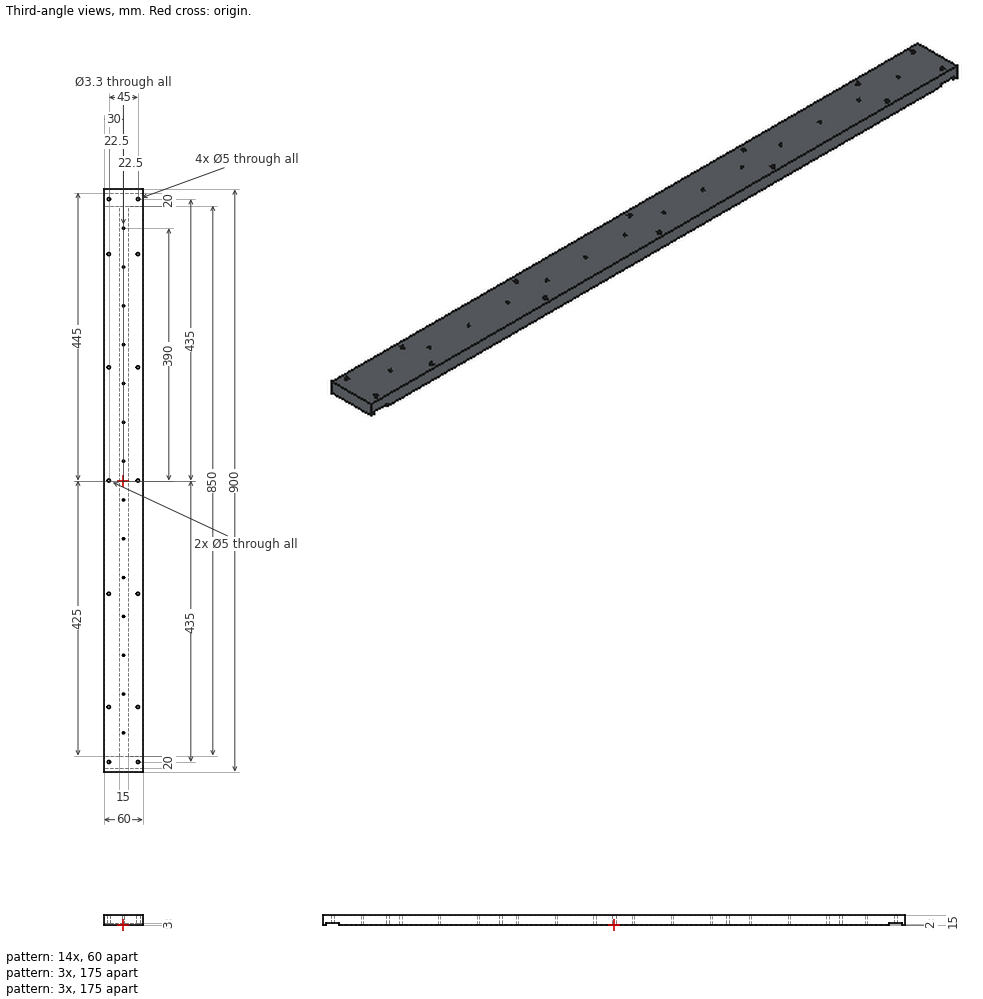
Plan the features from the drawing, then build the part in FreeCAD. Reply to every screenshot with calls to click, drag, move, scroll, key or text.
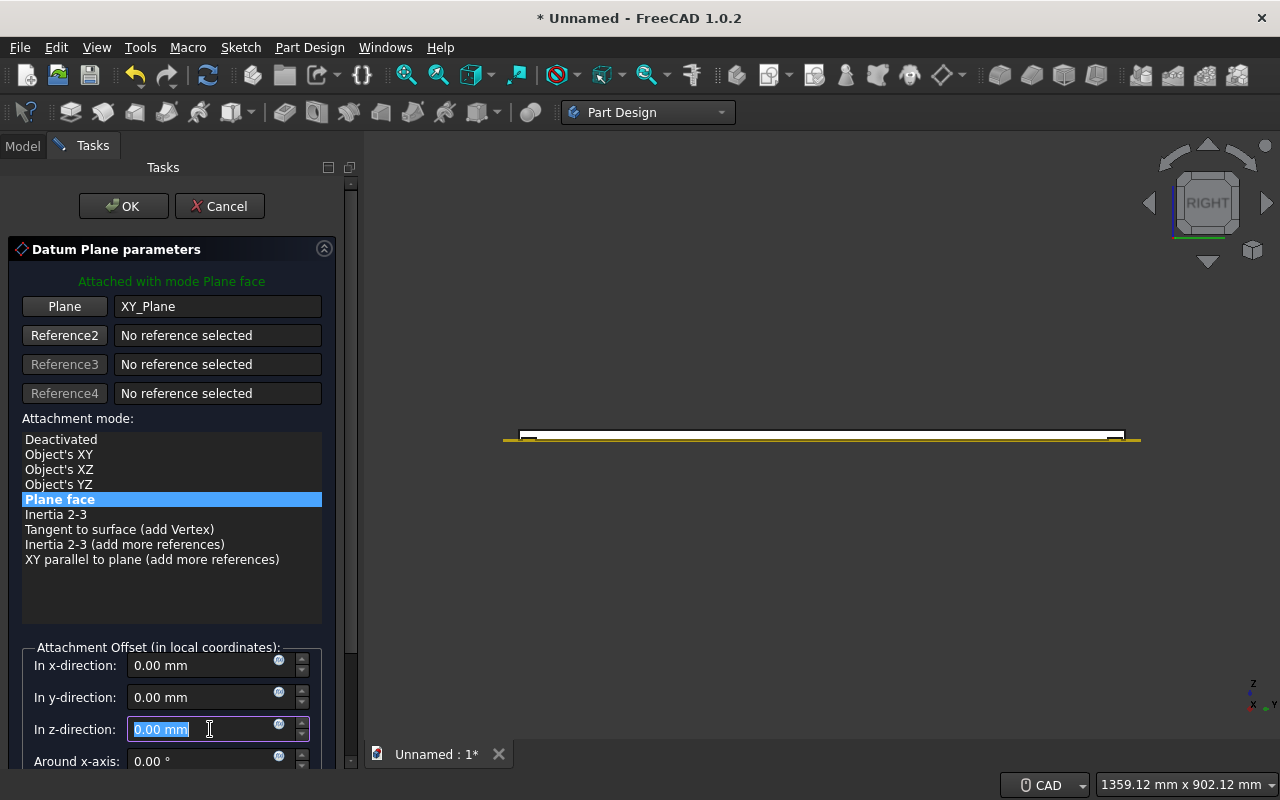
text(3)
key(Tab)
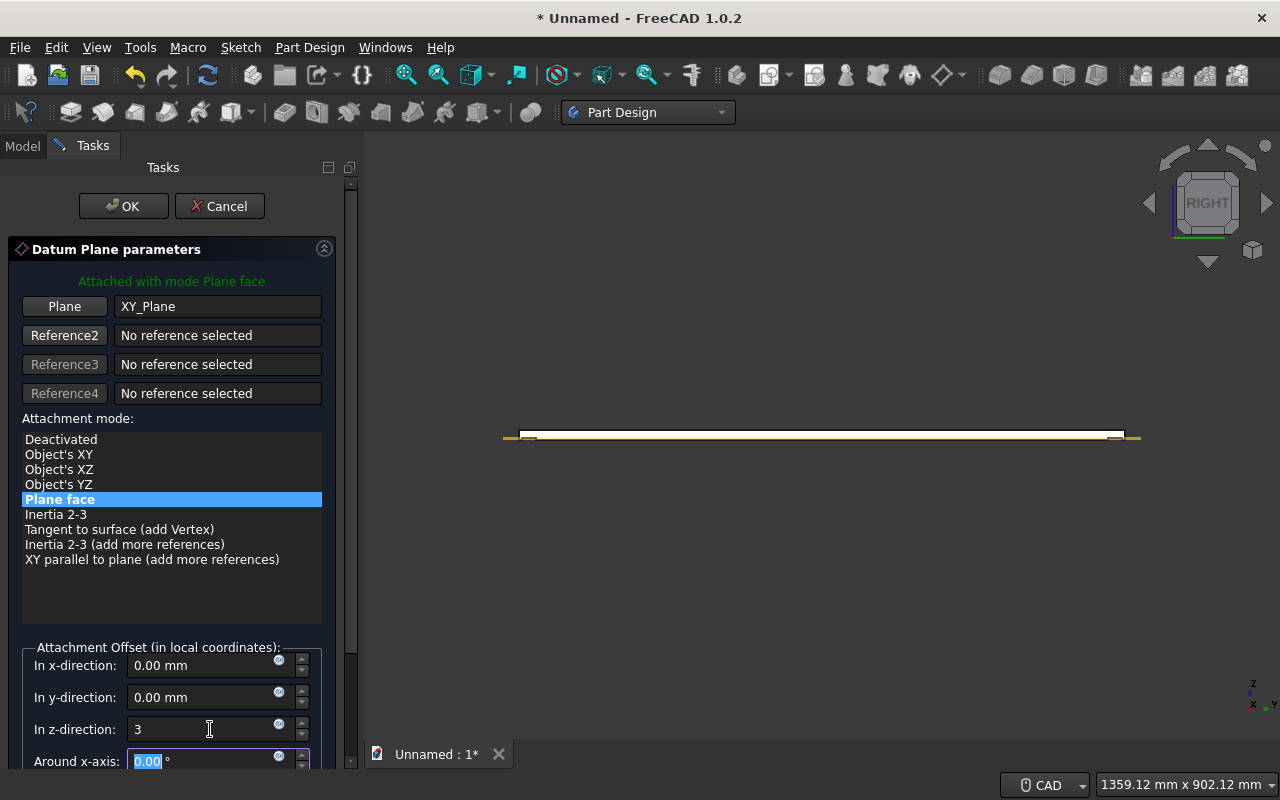
click(124, 206)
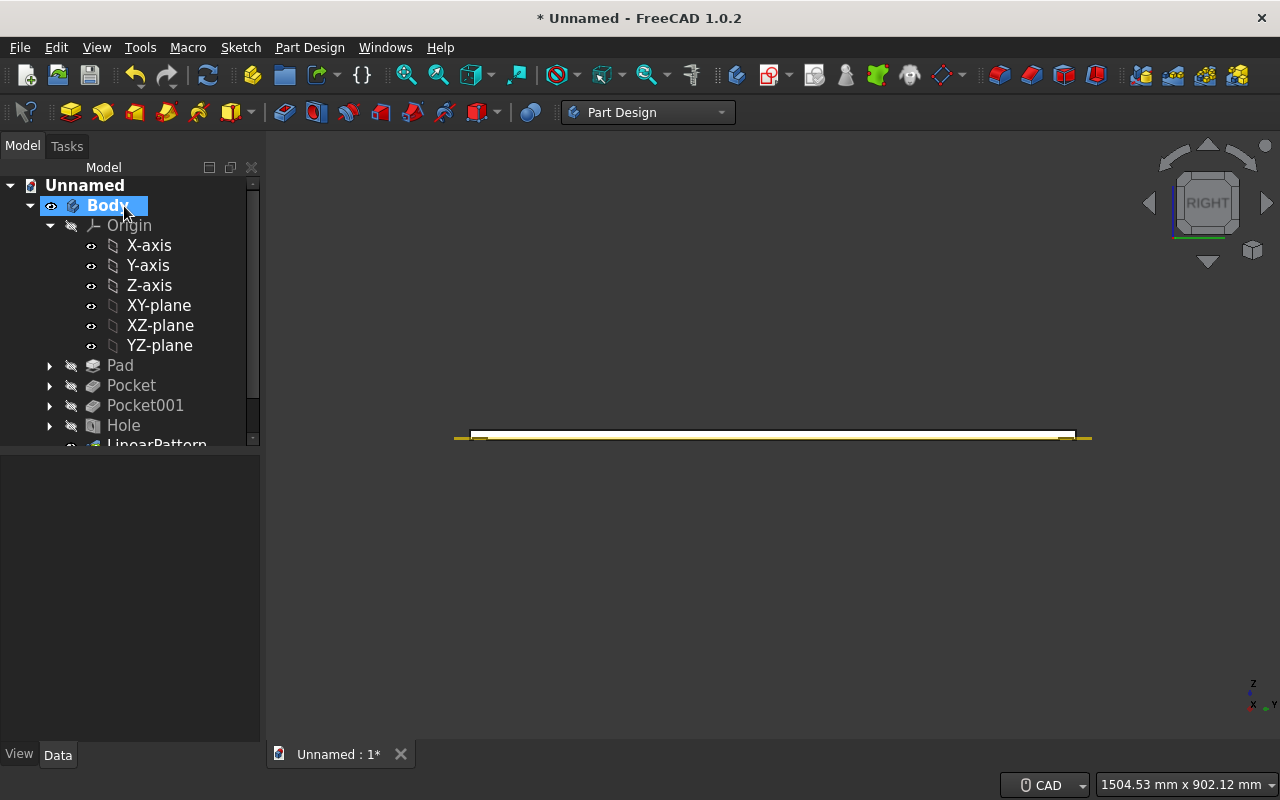
scroll(100, 321, down, 3)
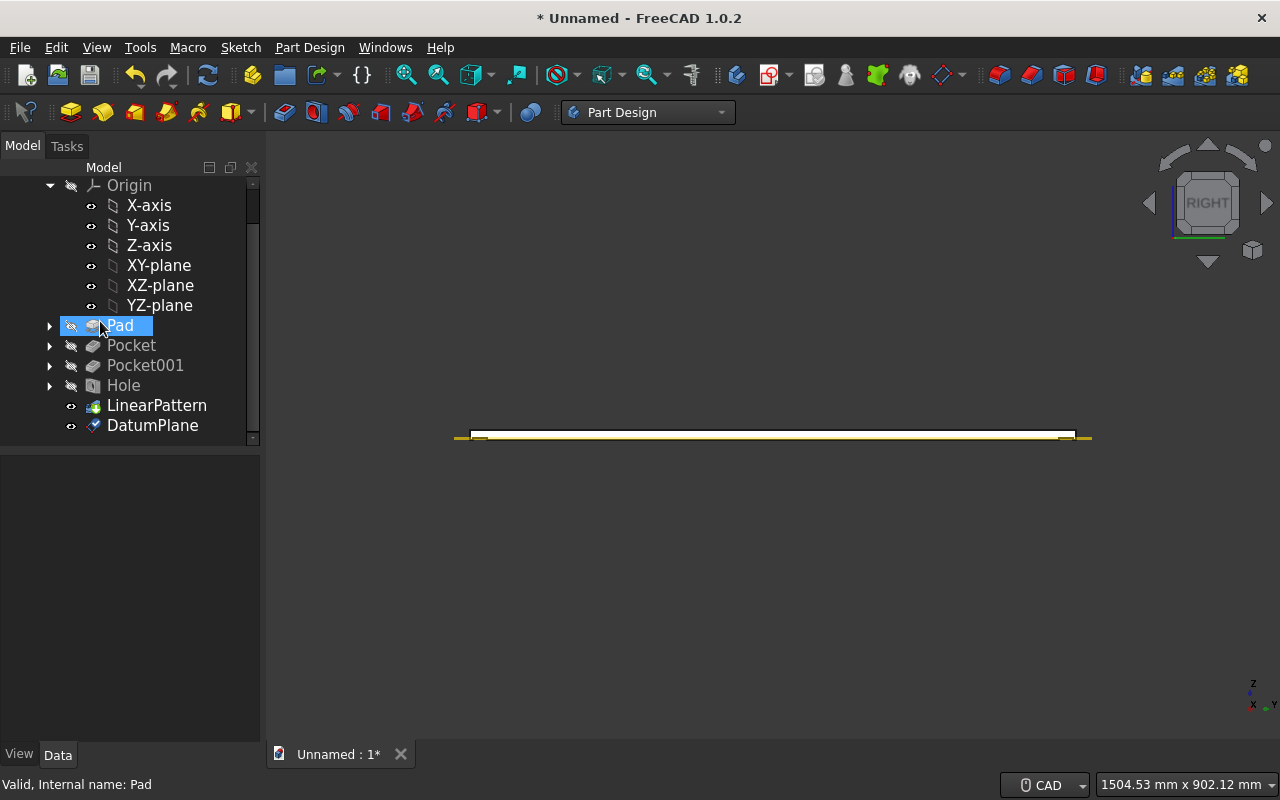
click(116, 426)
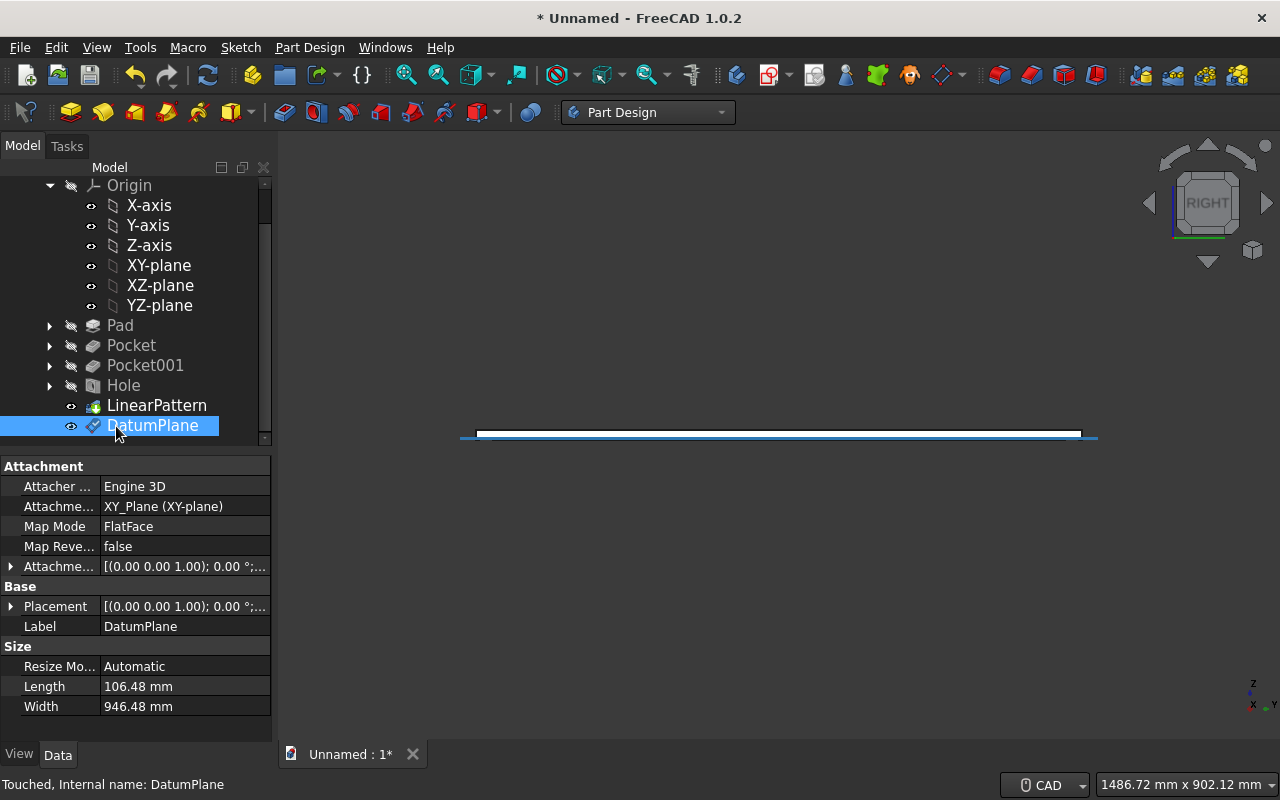
click(770, 76)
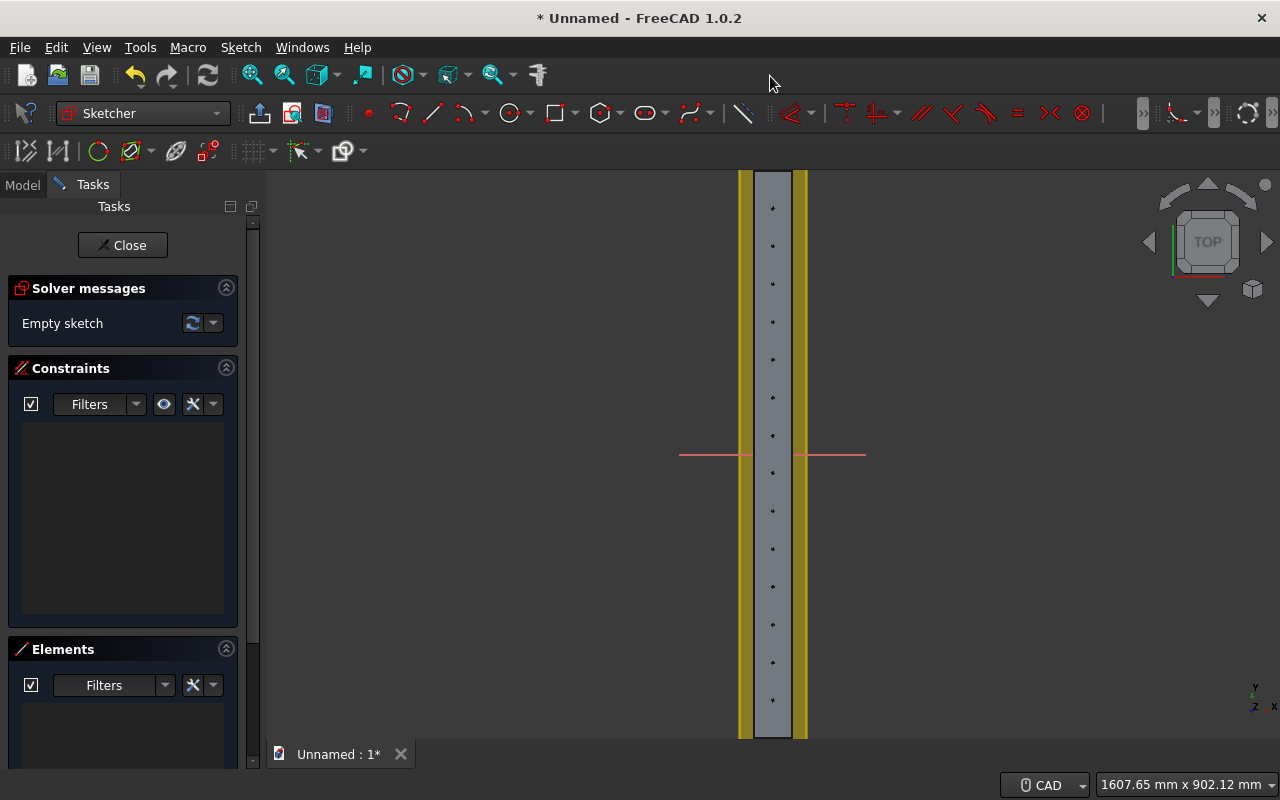
key(q)
key(s)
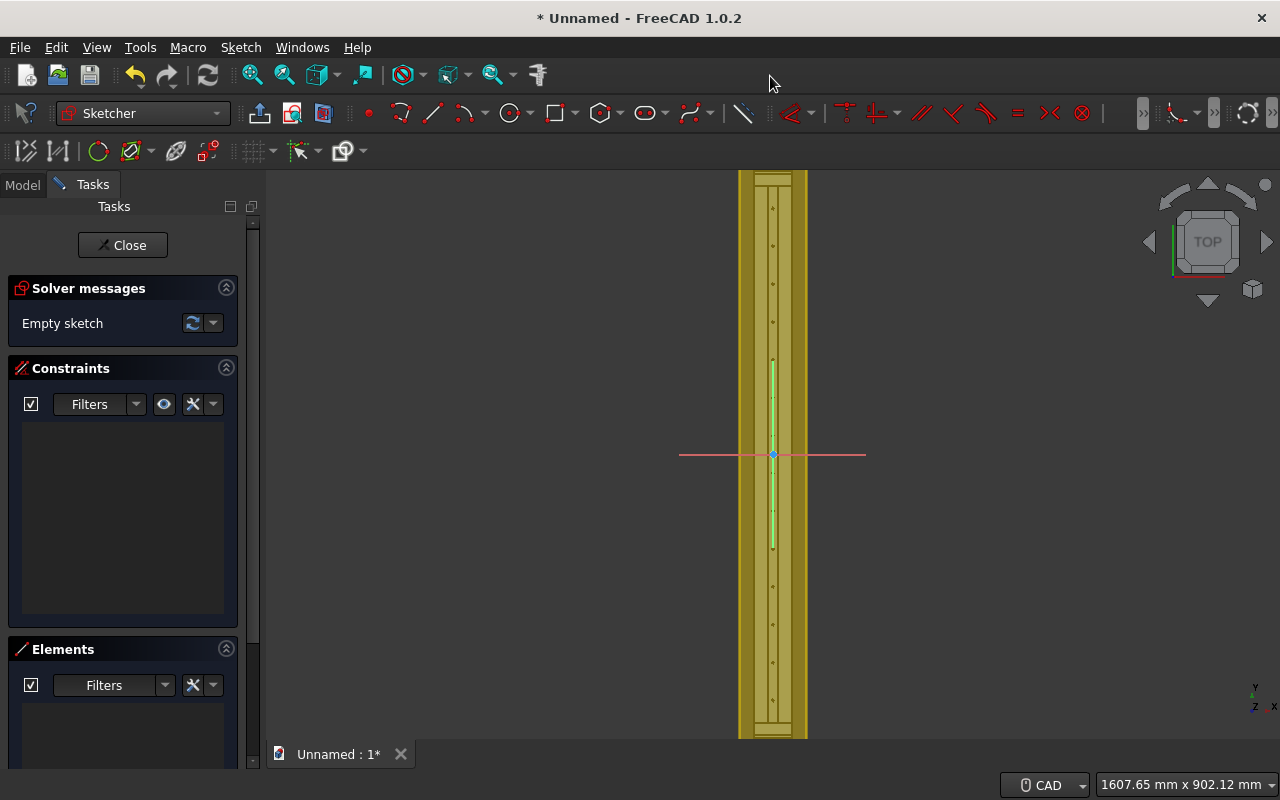
scroll(565, 455, down, 2)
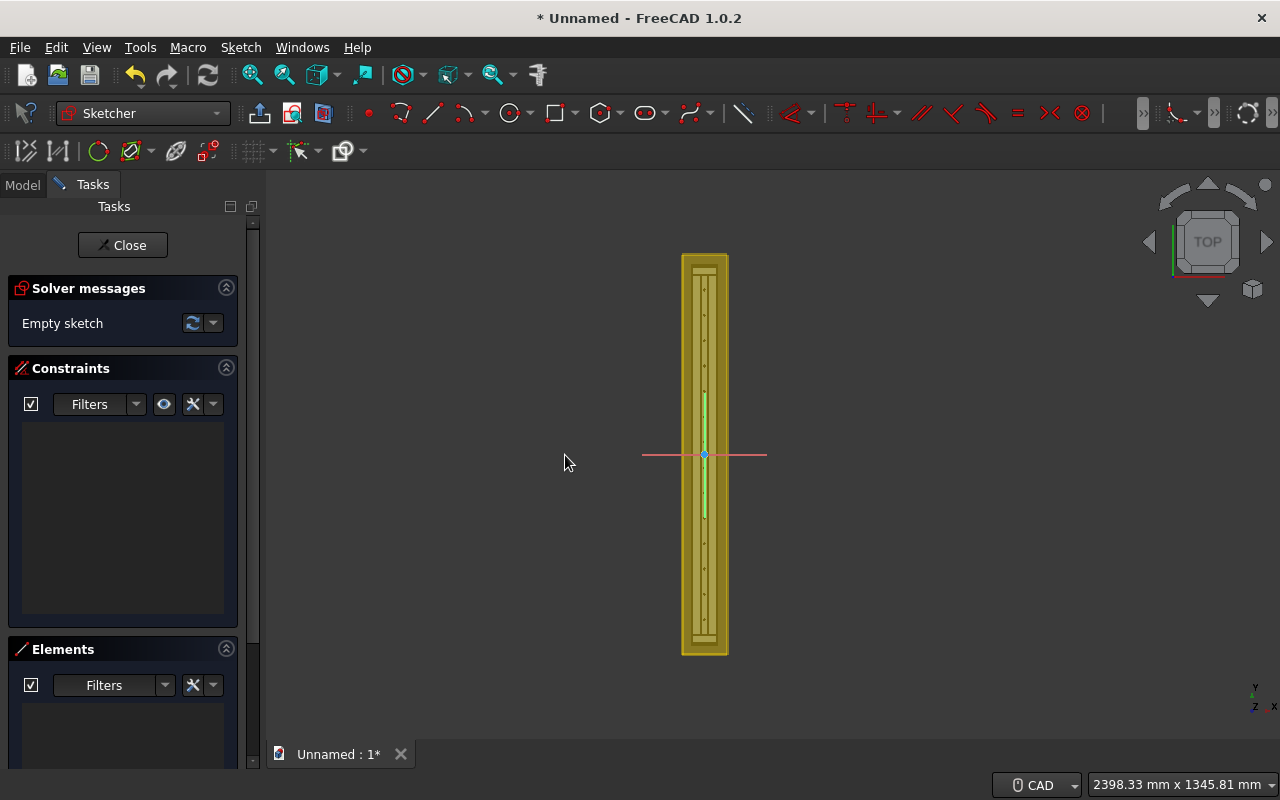
key(g)
key(c)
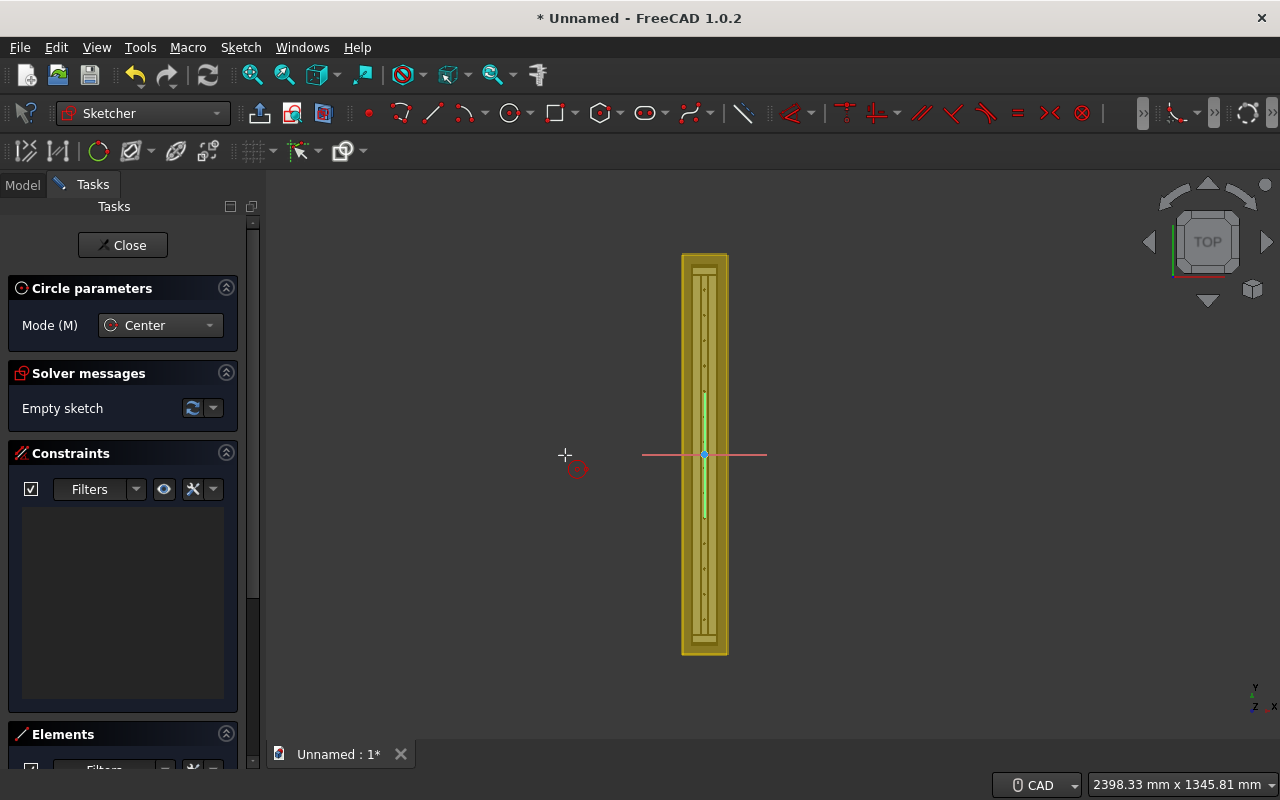
scroll(714, 271, up, 16)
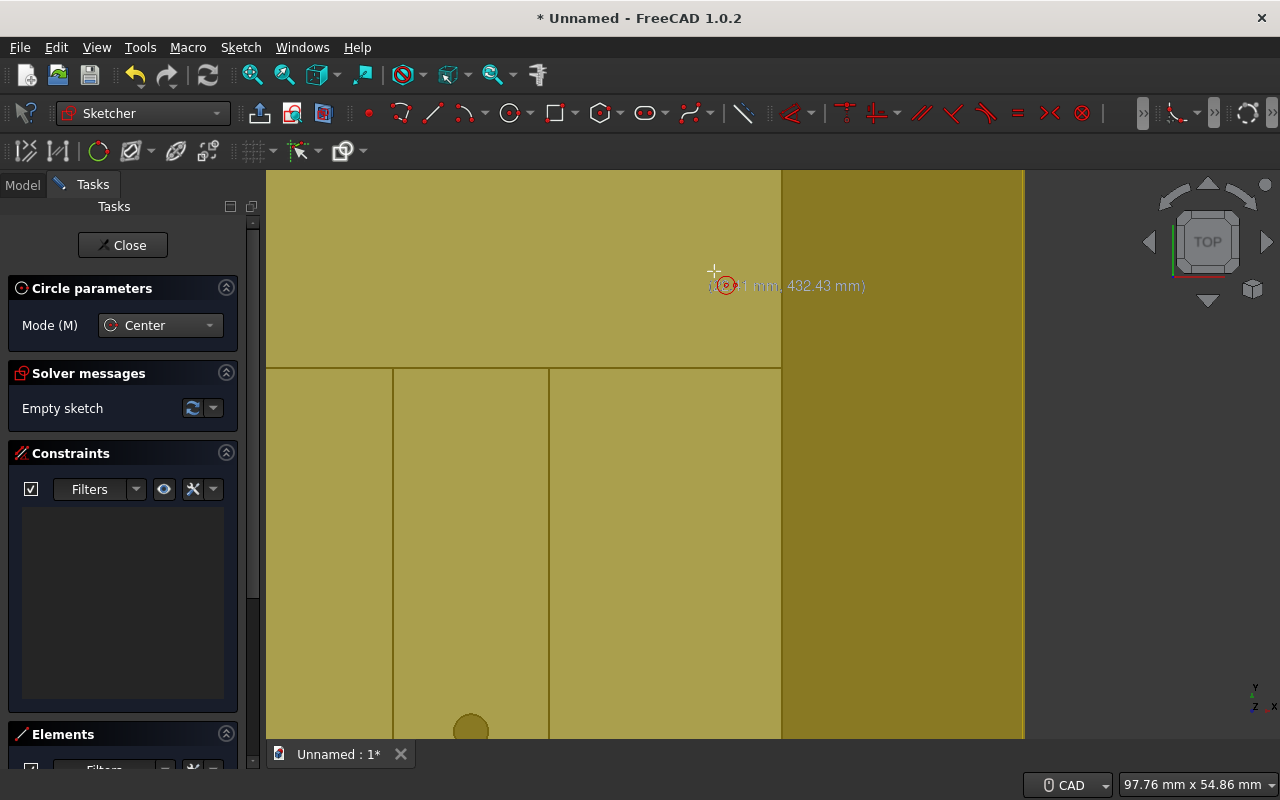
scroll(717, 228, down, 15)